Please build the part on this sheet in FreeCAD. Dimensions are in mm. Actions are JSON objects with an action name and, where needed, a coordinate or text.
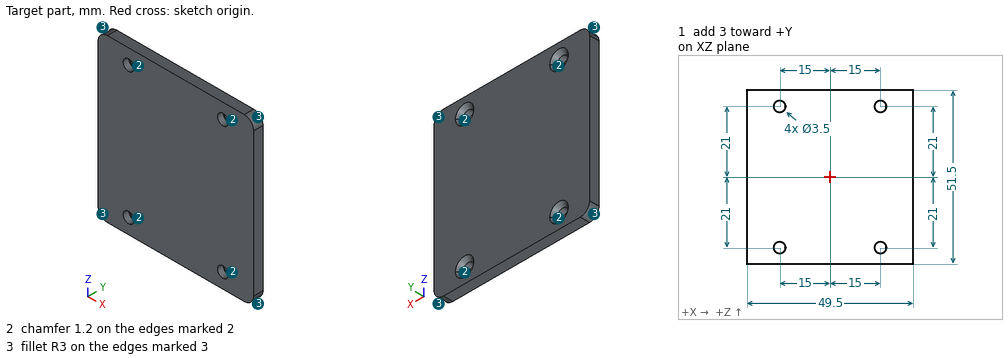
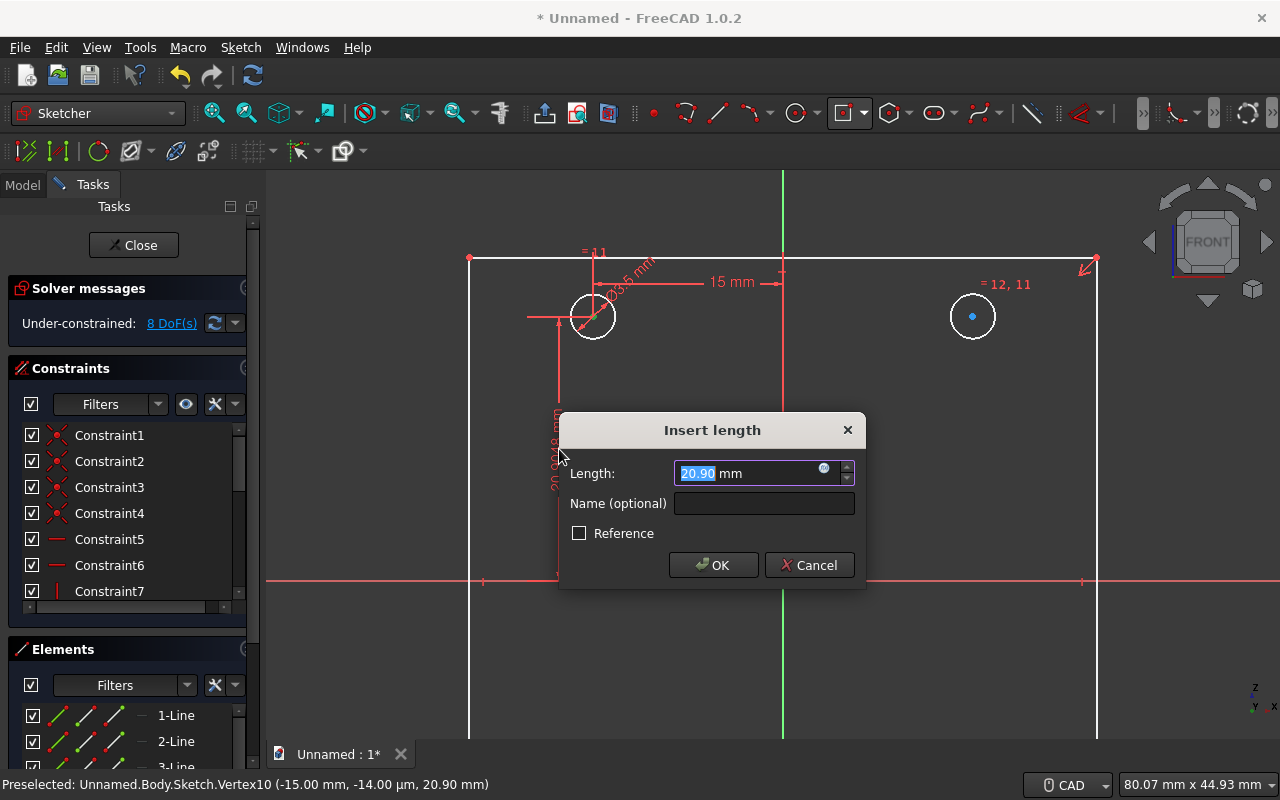
{"action": "type", "text": "21"}
{"action": "key", "text": "Return"}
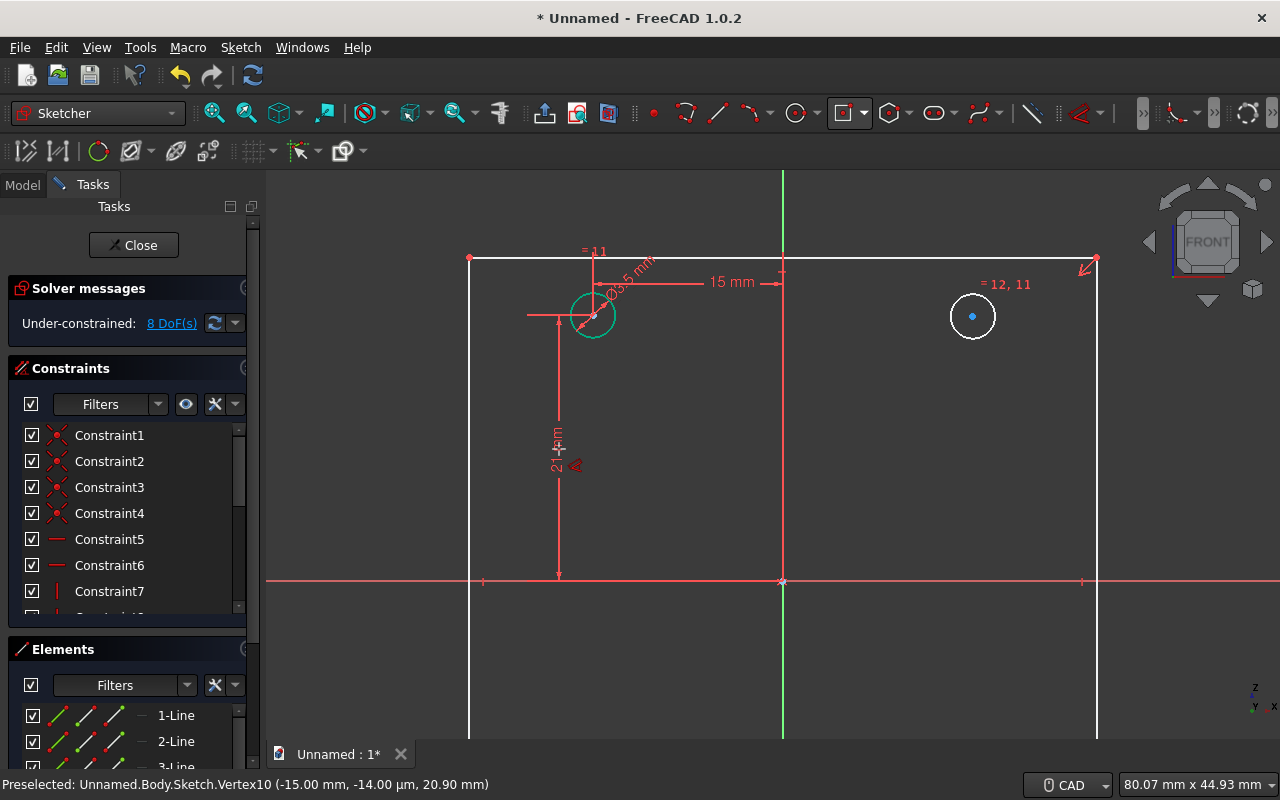
{"action": "left_click", "coordinate": [973, 316]}
{"action": "left_click", "coordinate": [878, 282]}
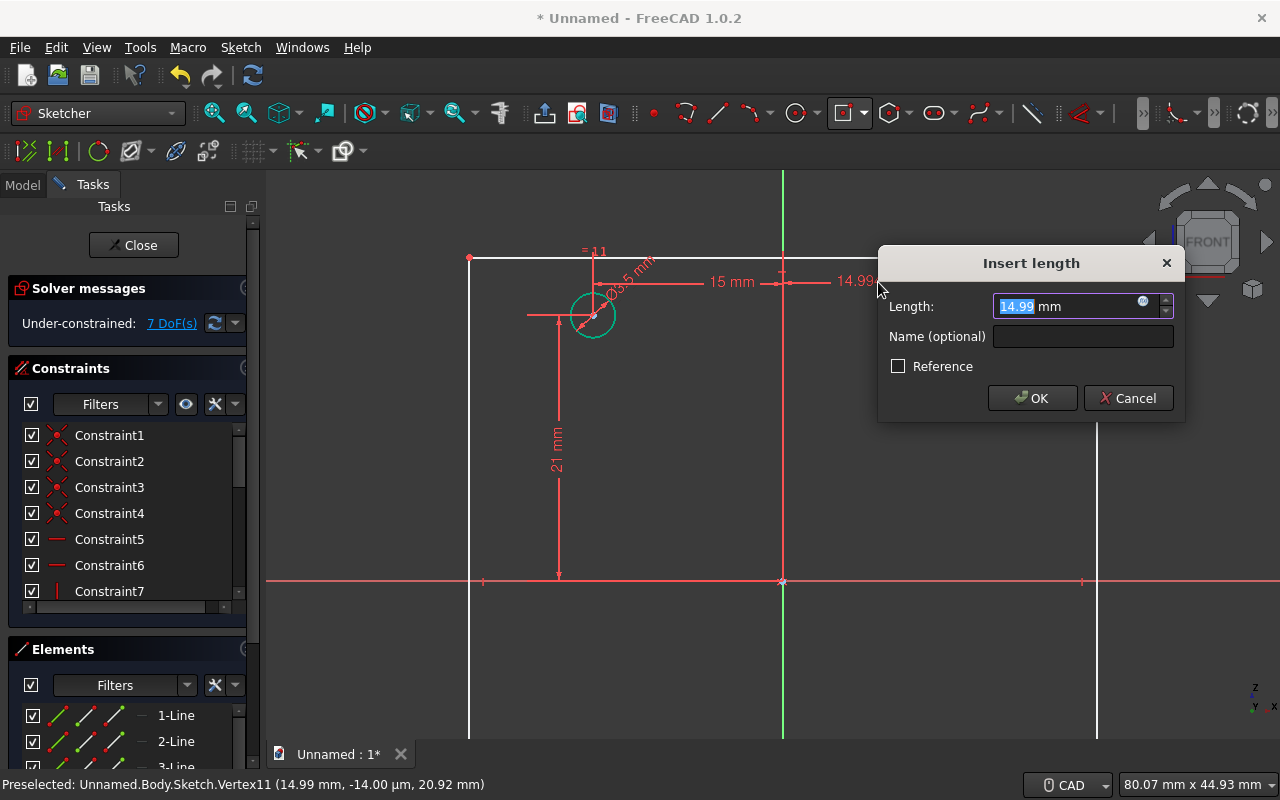
{"action": "type", "text": "15"}
{"action": "key", "text": "Return"}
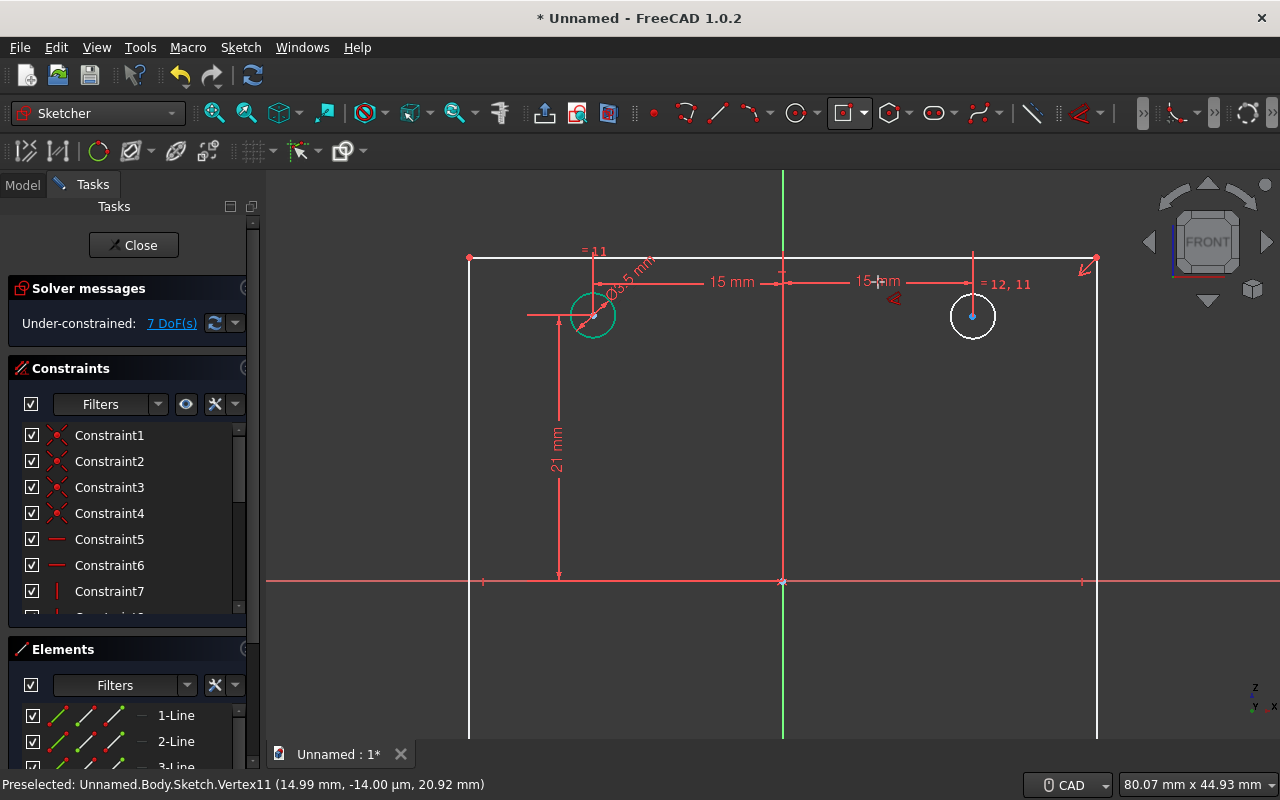
{"action": "left_click", "coordinate": [973, 316]}
{"action": "left_click", "coordinate": [1007, 449]}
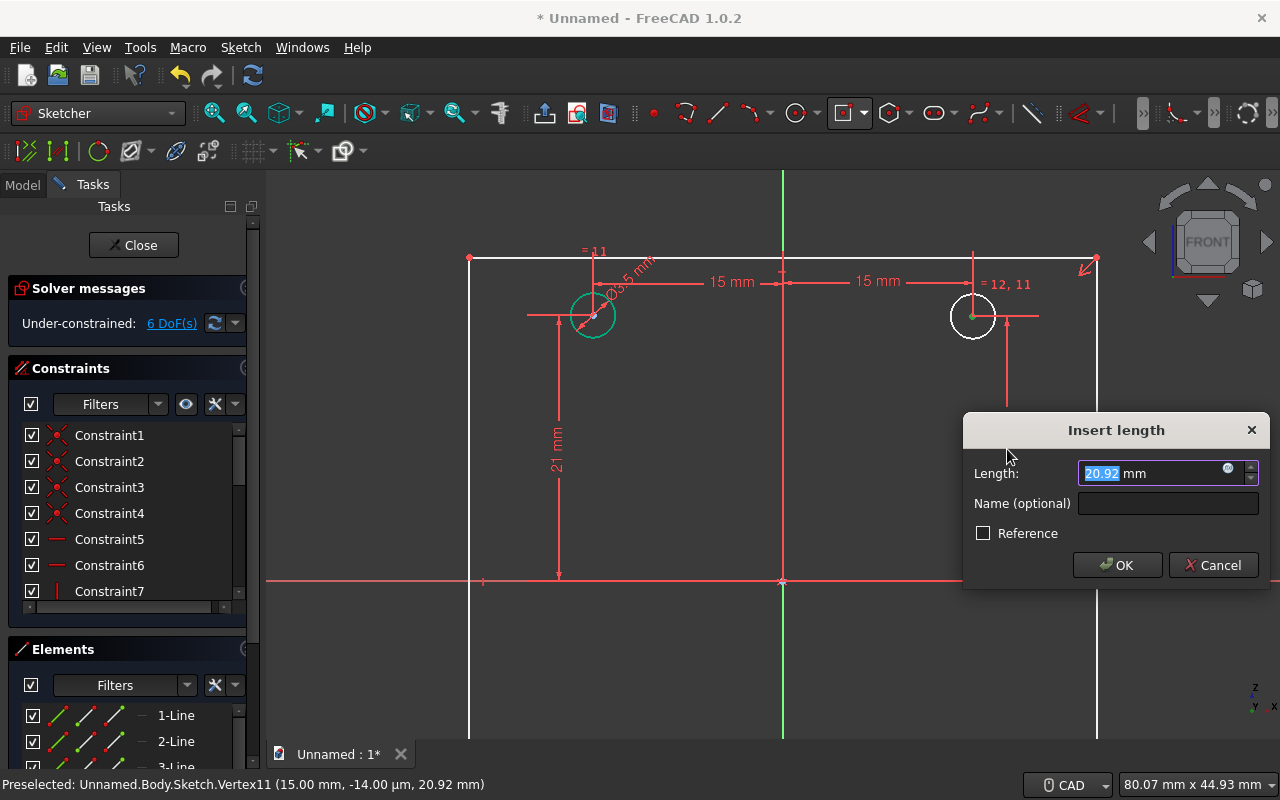
{"action": "type", "text": "21"}
{"action": "key", "text": "Return"}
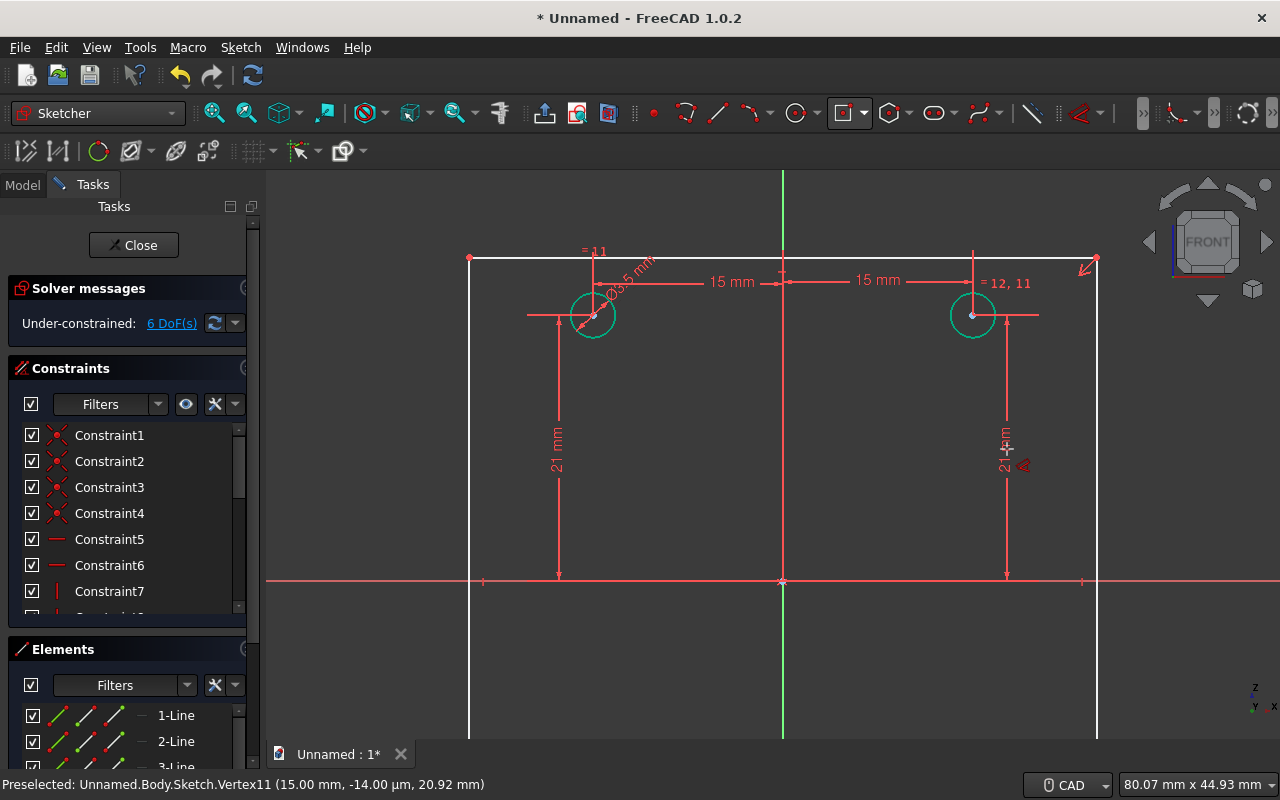
{"action": "scroll", "coordinate": [609, 300], "scroll_direction": "down", "scroll_amount": 3}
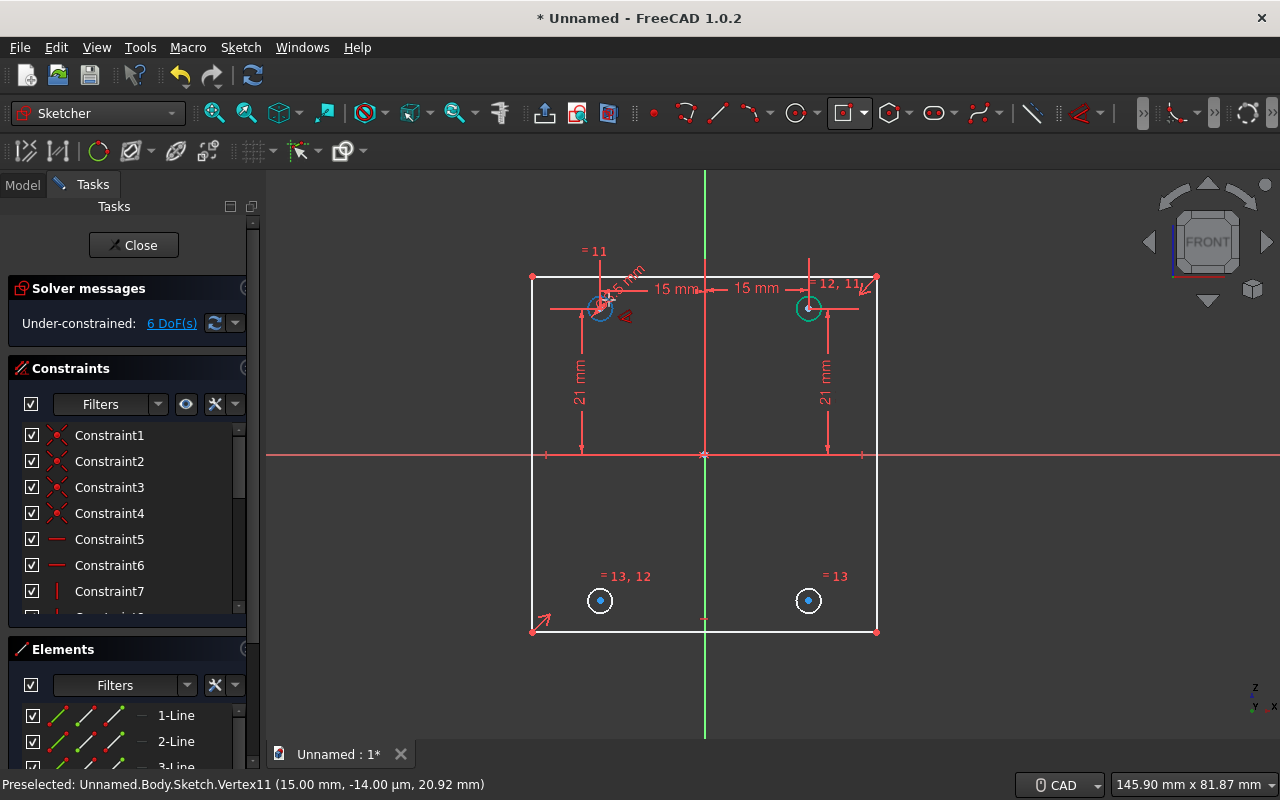
{"action": "left_click", "coordinate": [600, 601]}
{"action": "left_click", "coordinate": [652, 421]}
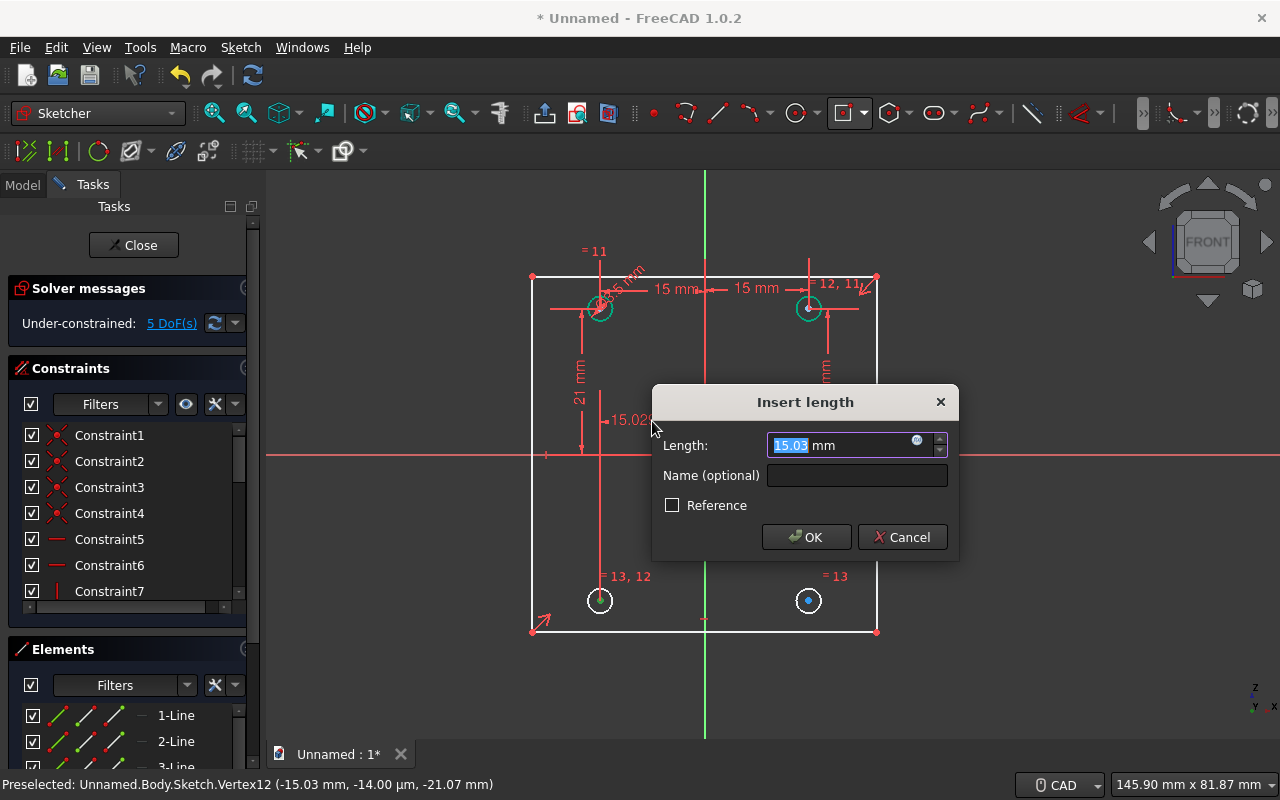
{"action": "type", "text": "15"}
{"action": "key", "text": "Return"}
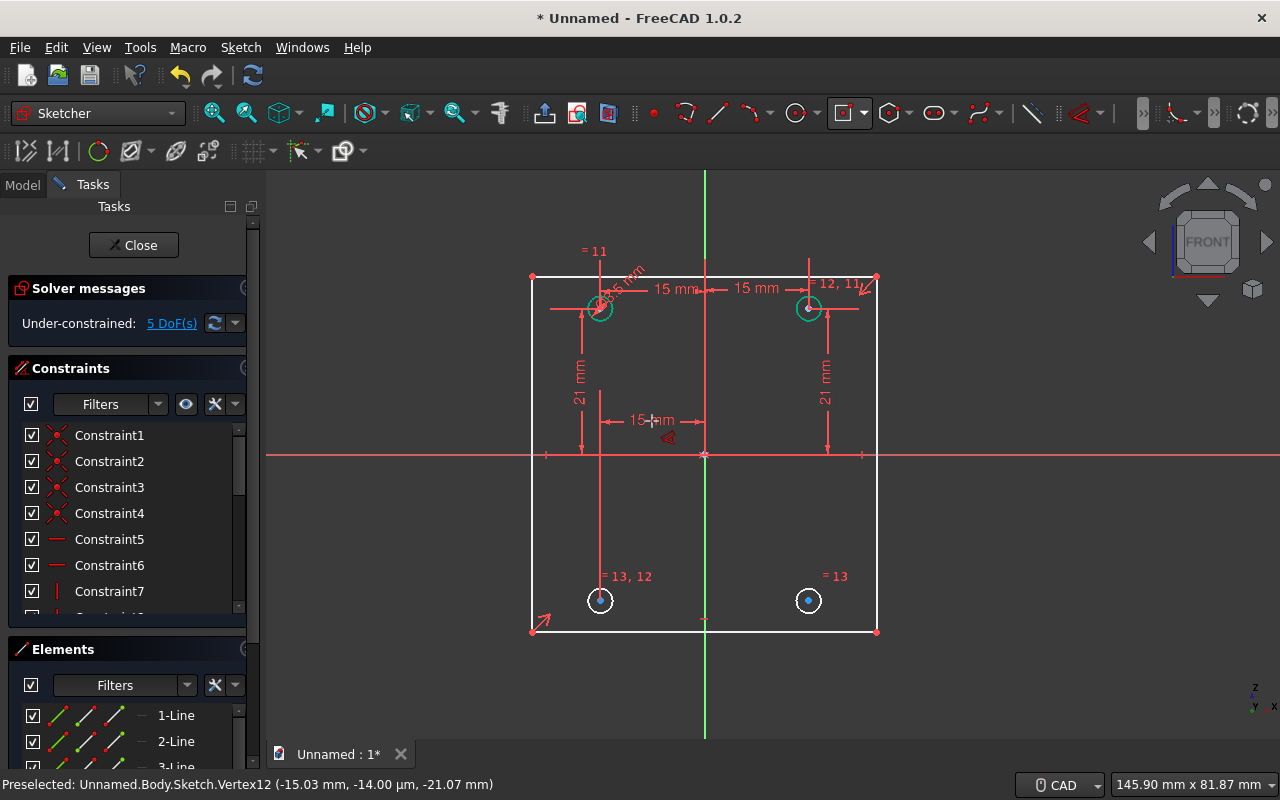
{"action": "left_click", "coordinate": [600, 601]}
{"action": "left_click", "coordinate": [566, 528]}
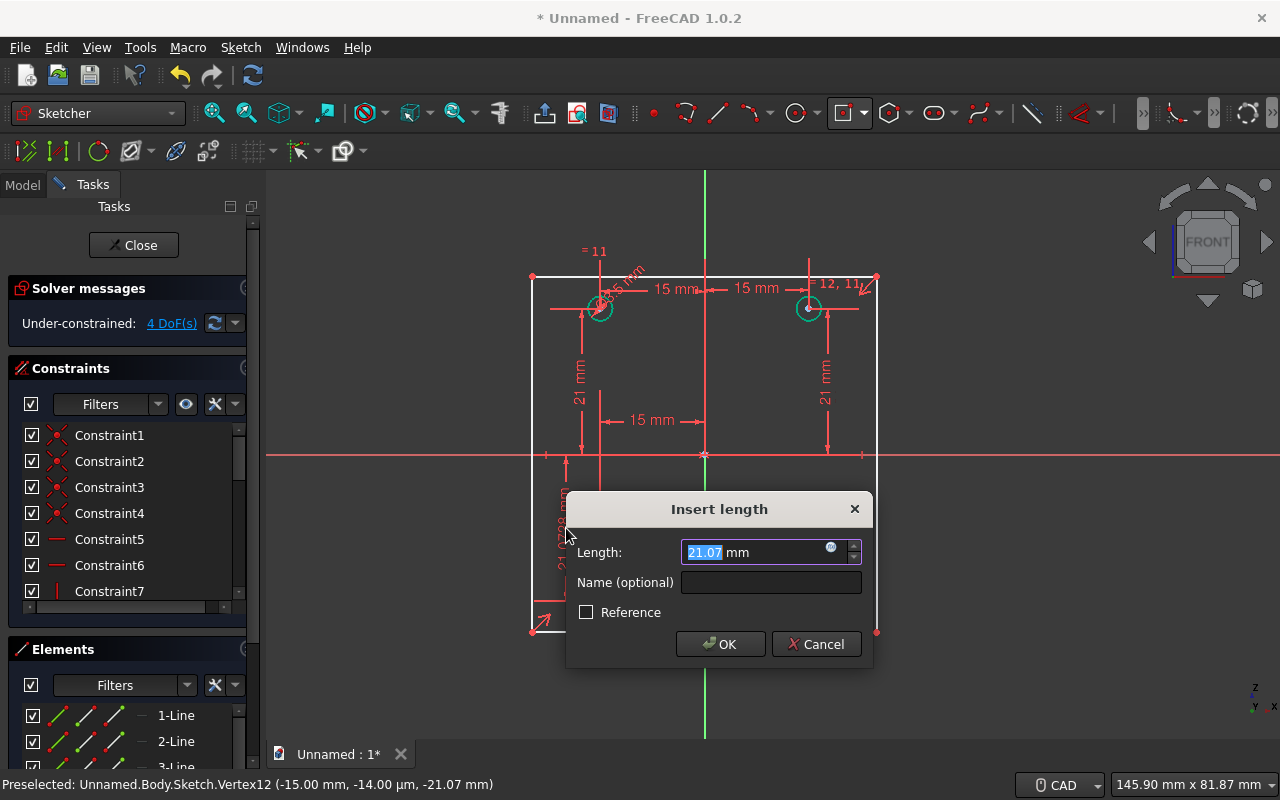
{"action": "type", "text": "21"}
{"action": "key", "text": "Return"}